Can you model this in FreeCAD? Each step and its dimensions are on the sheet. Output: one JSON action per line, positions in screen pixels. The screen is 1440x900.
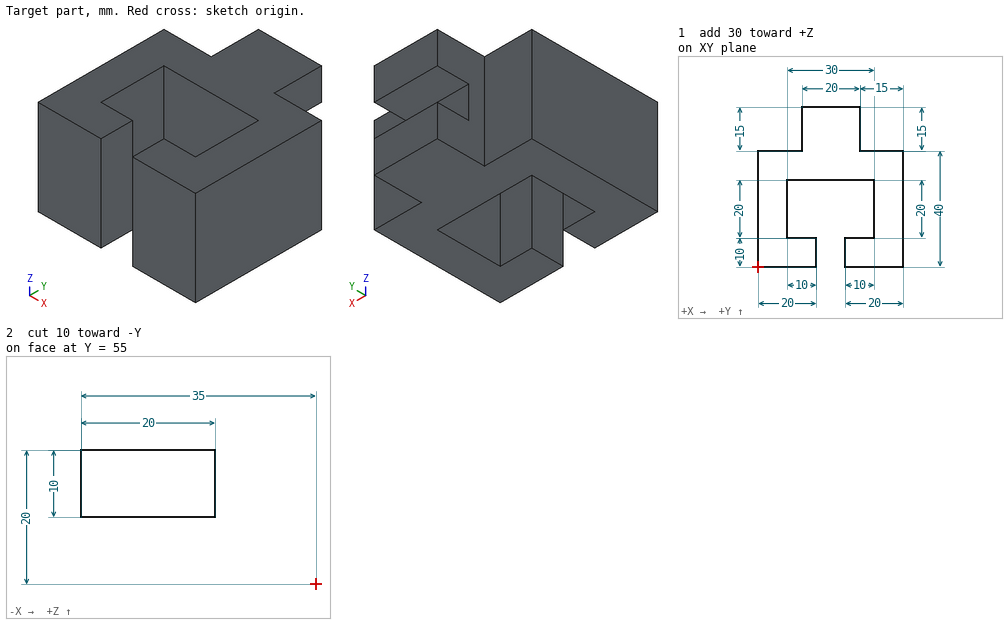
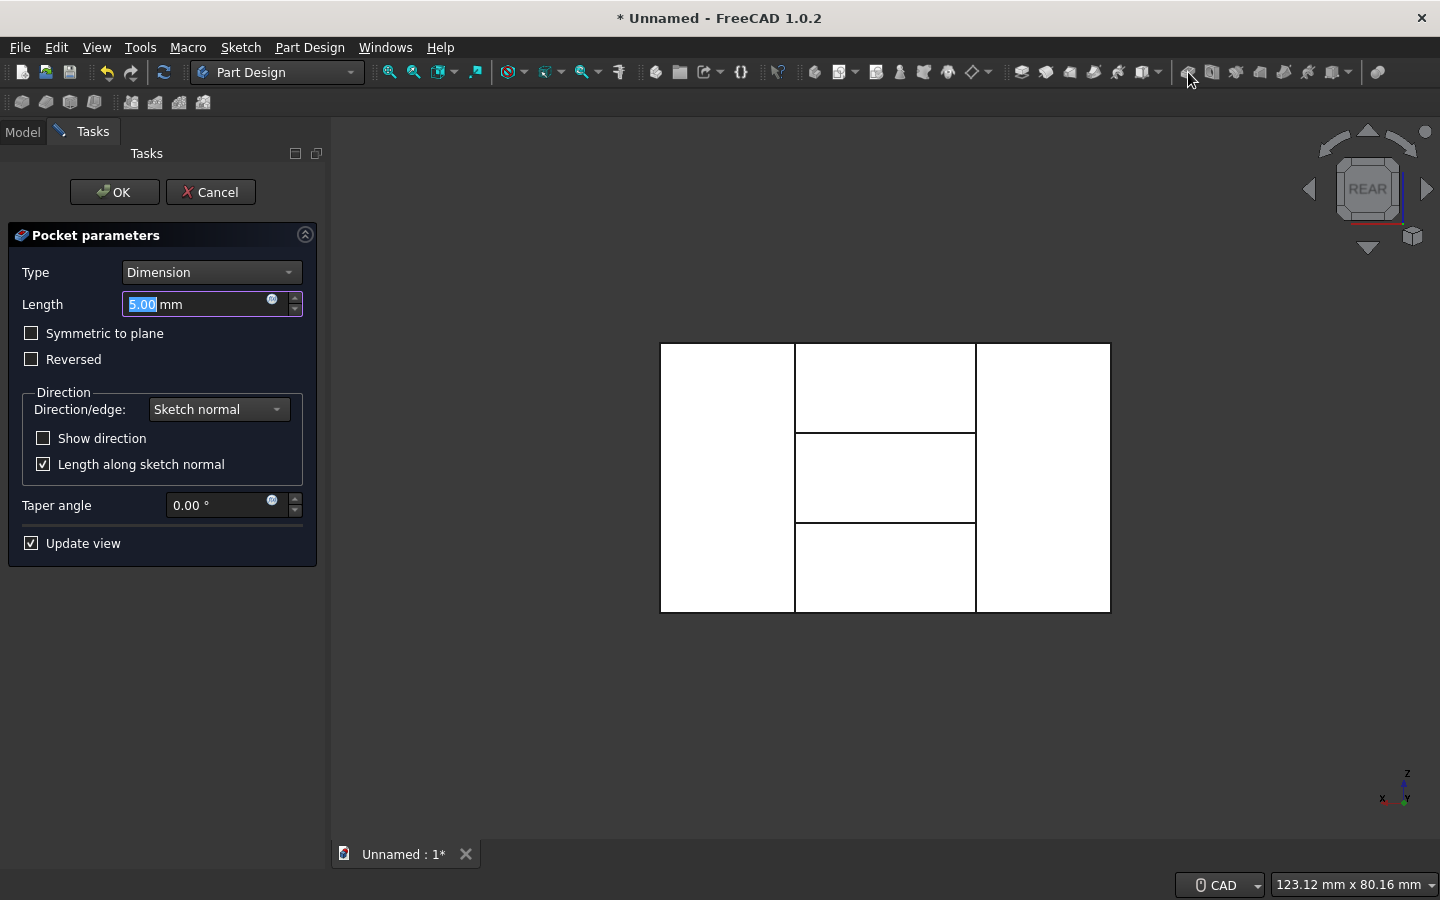
{"action": "type", "text": "10"}
{"action": "key", "text": "Tab"}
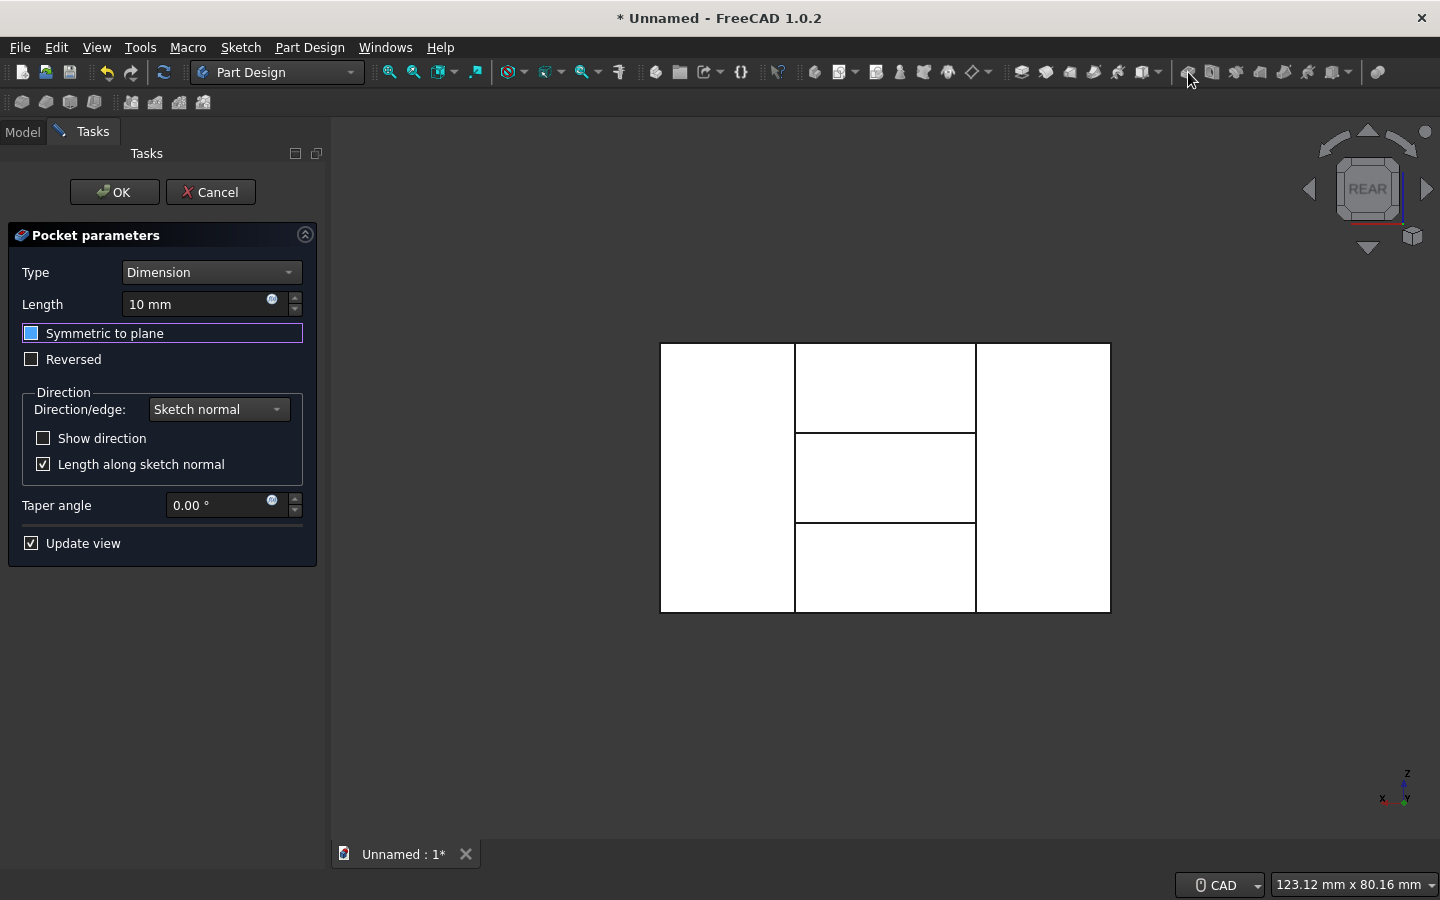
{"action": "left_click", "coordinate": [115, 192]}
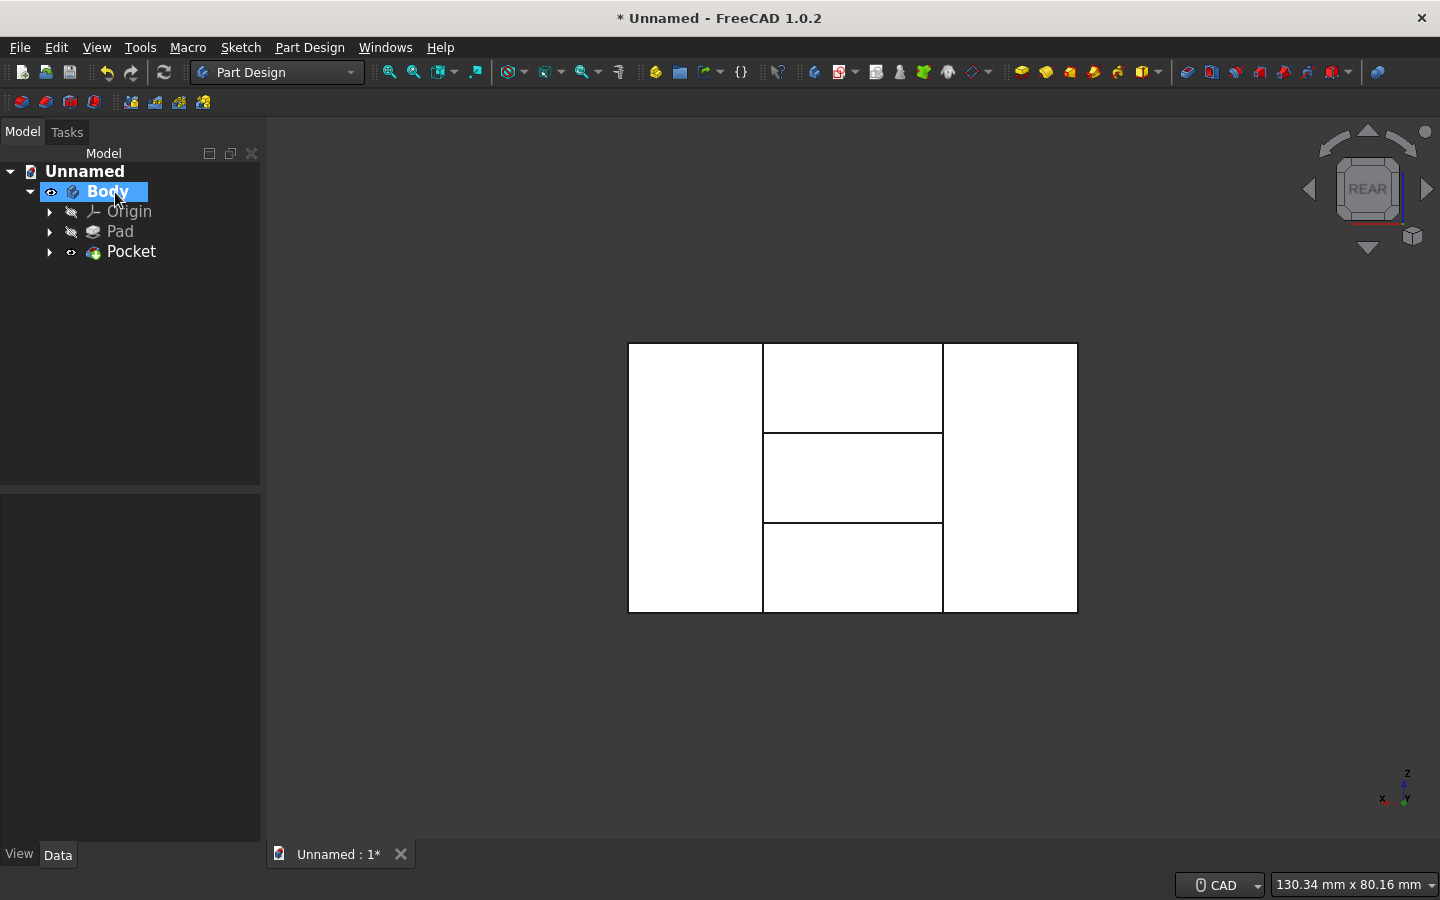
{"action": "key", "text": "0"}